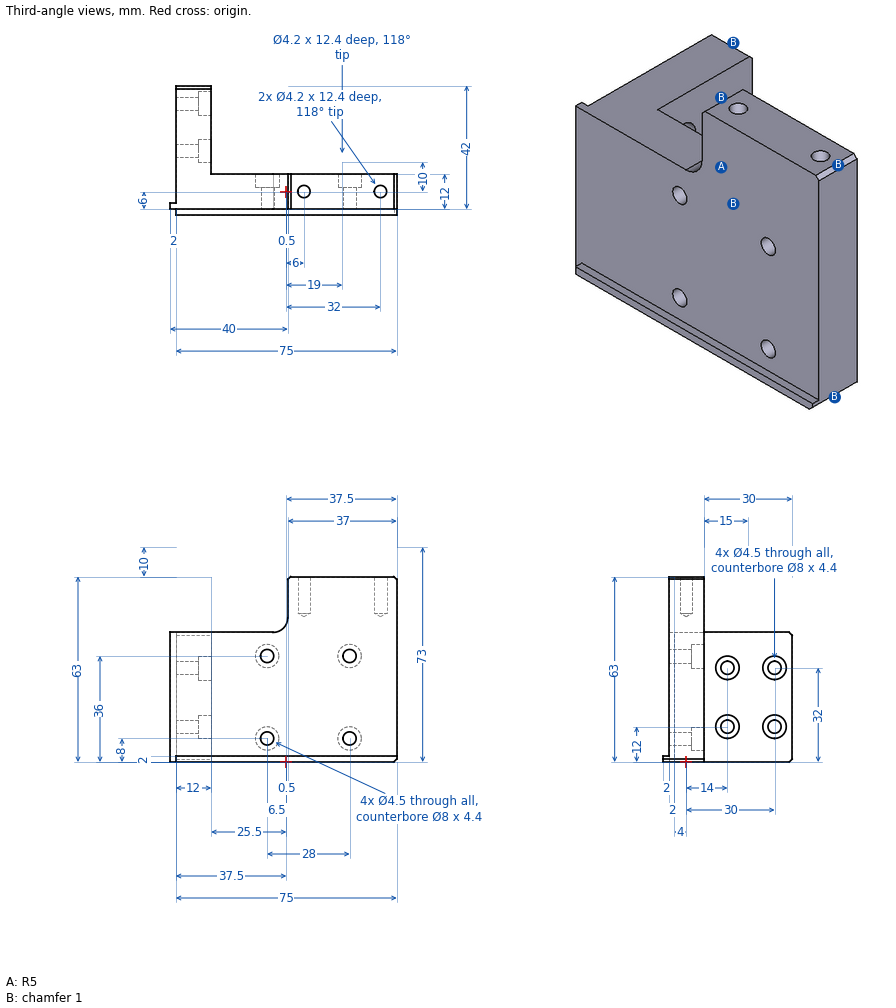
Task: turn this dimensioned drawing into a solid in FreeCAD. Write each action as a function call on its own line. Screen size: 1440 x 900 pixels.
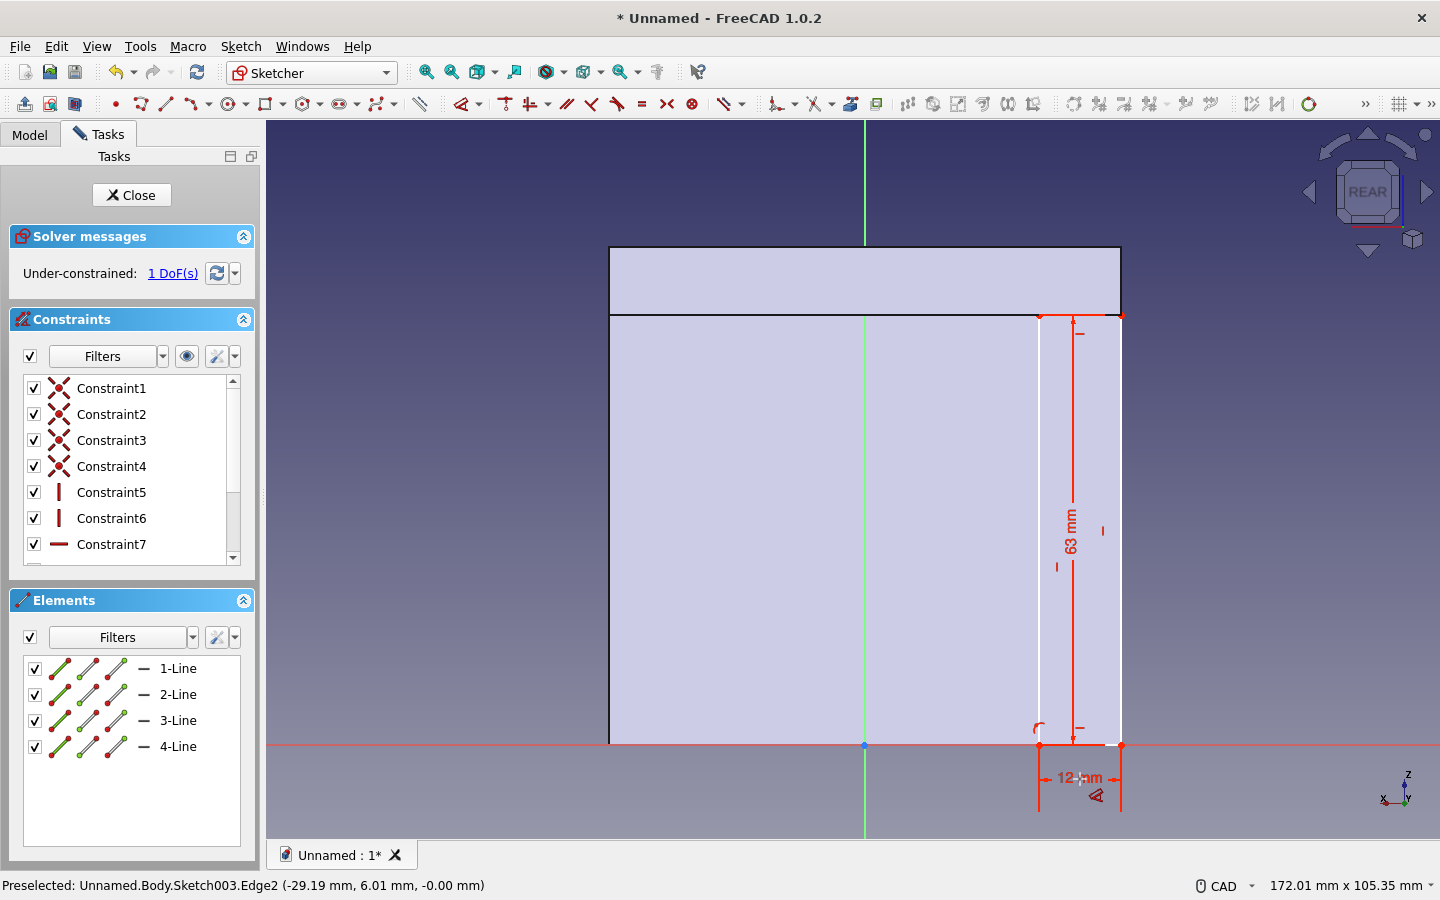
click(1039, 315)
click(952, 779)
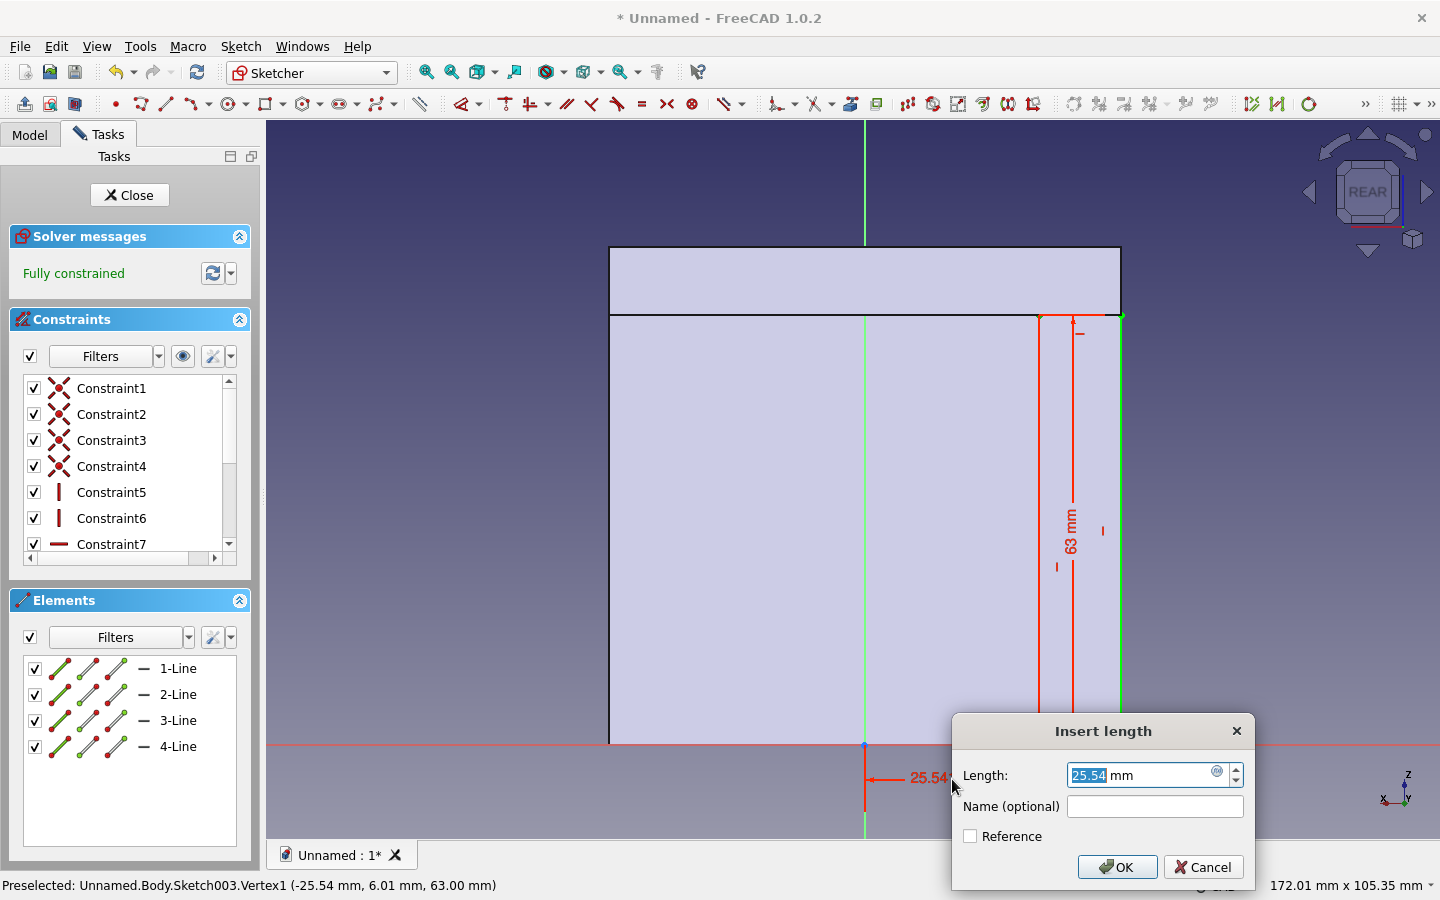
text(25.5)
key(Return)
key(Escape)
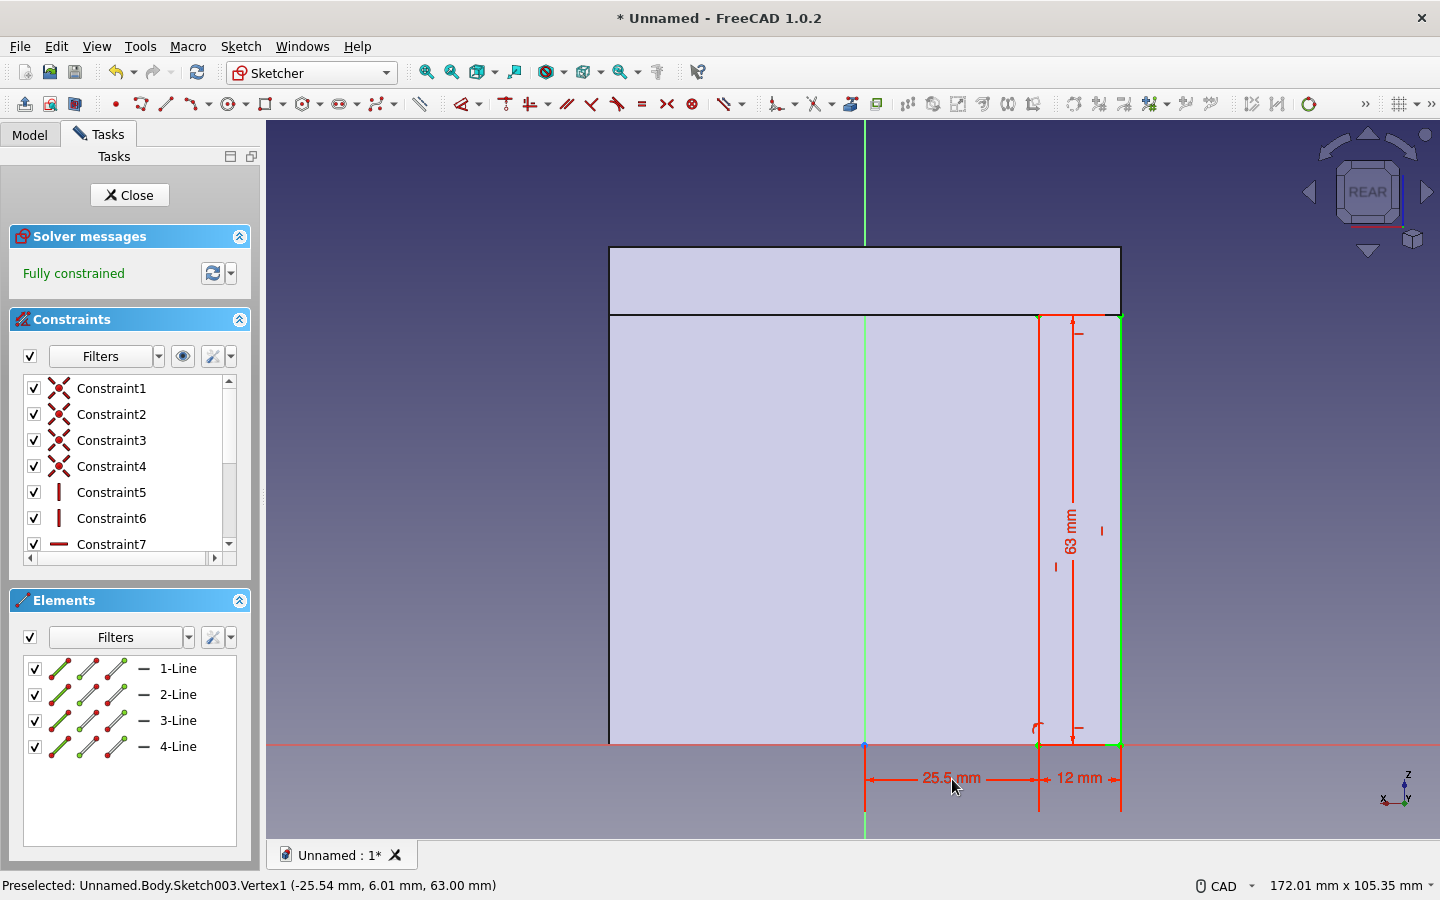
click(130, 195)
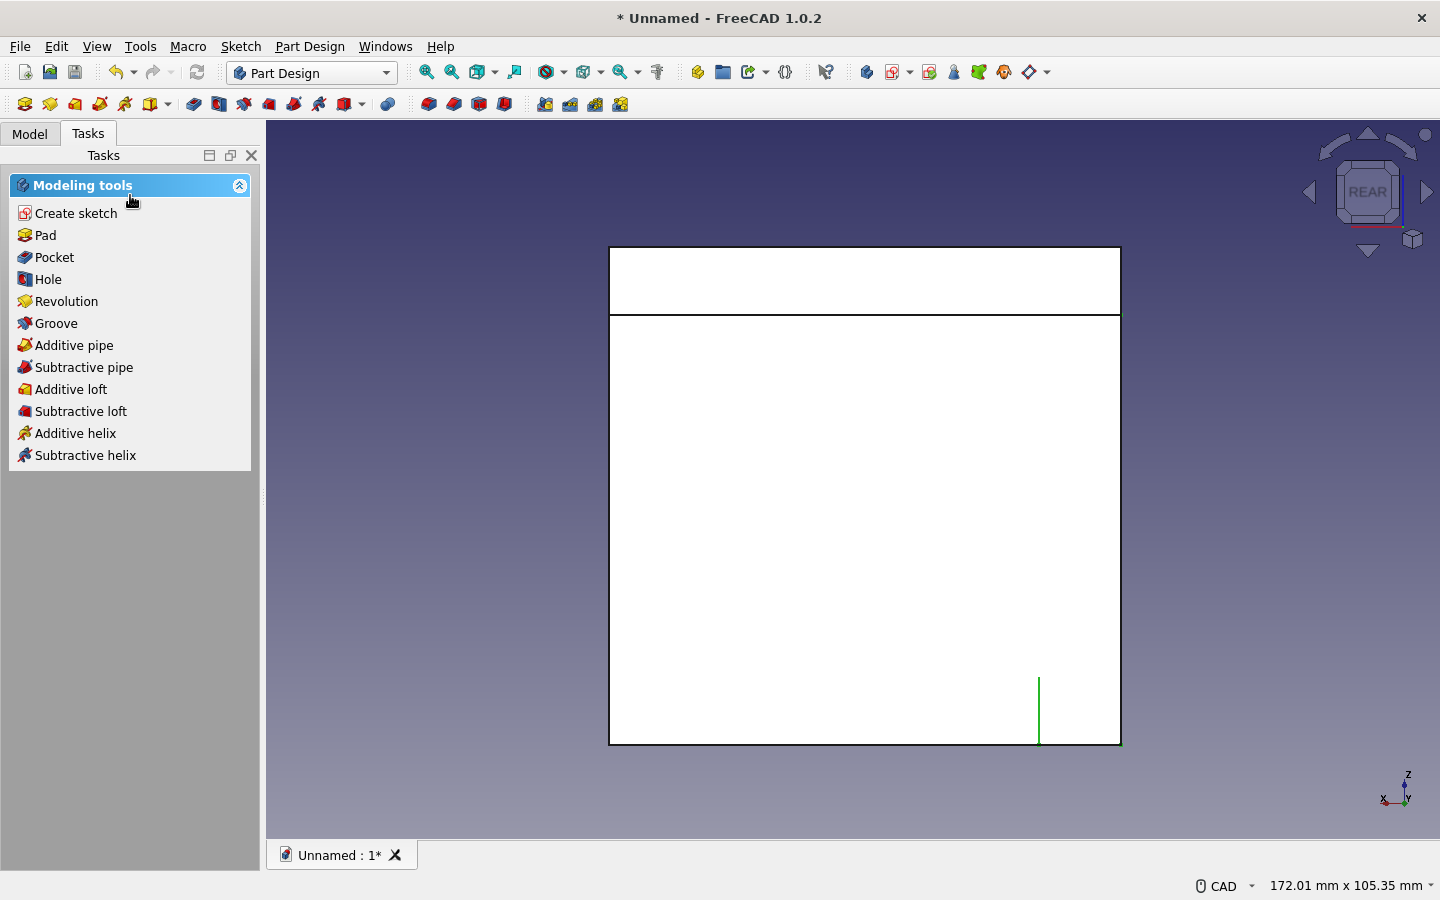
click(25, 104)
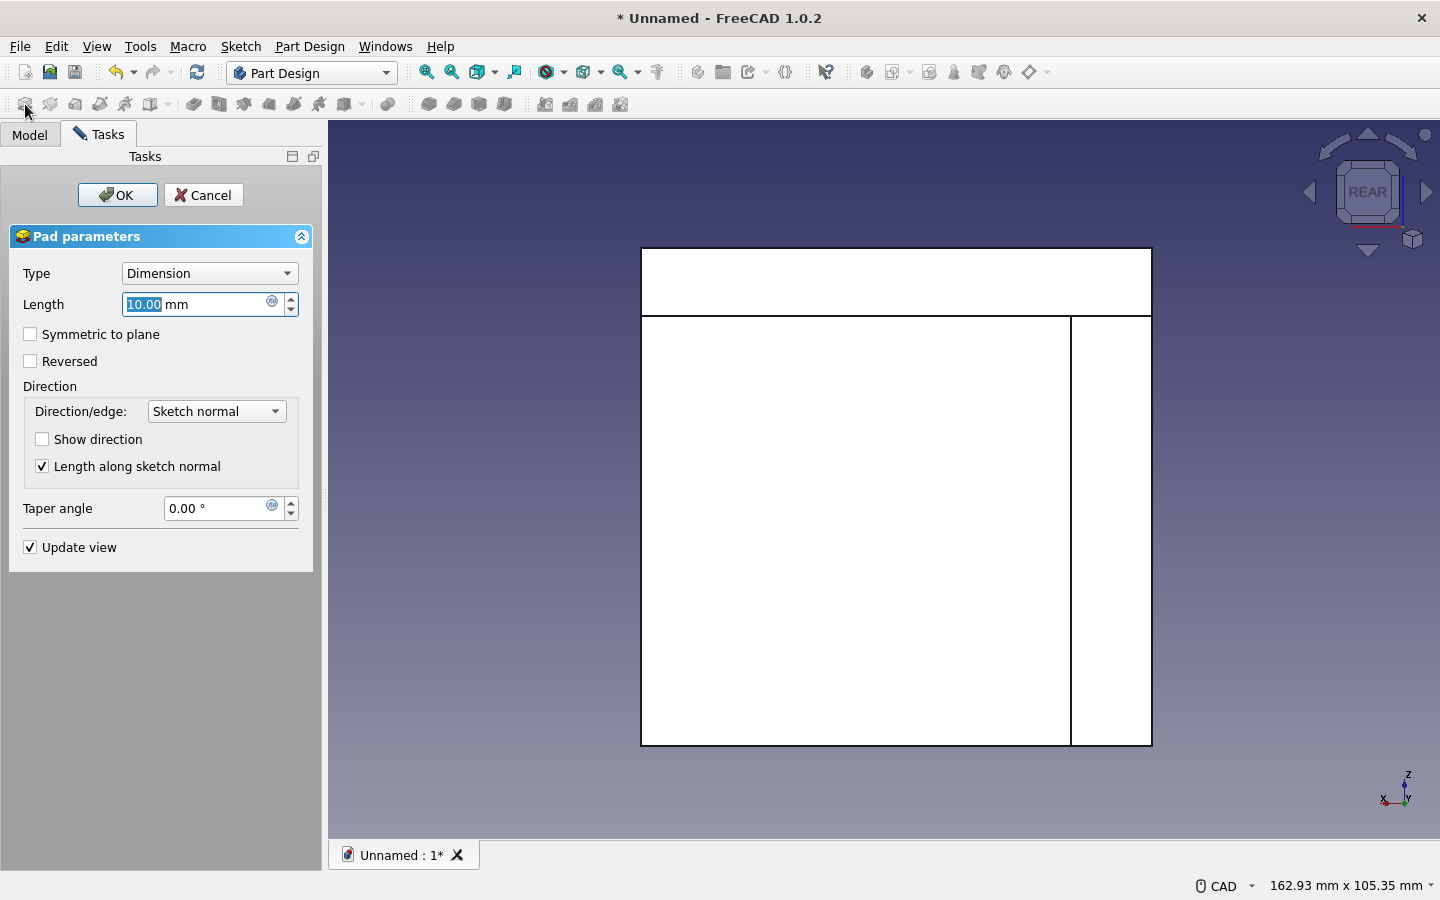
text(30)
key(Tab)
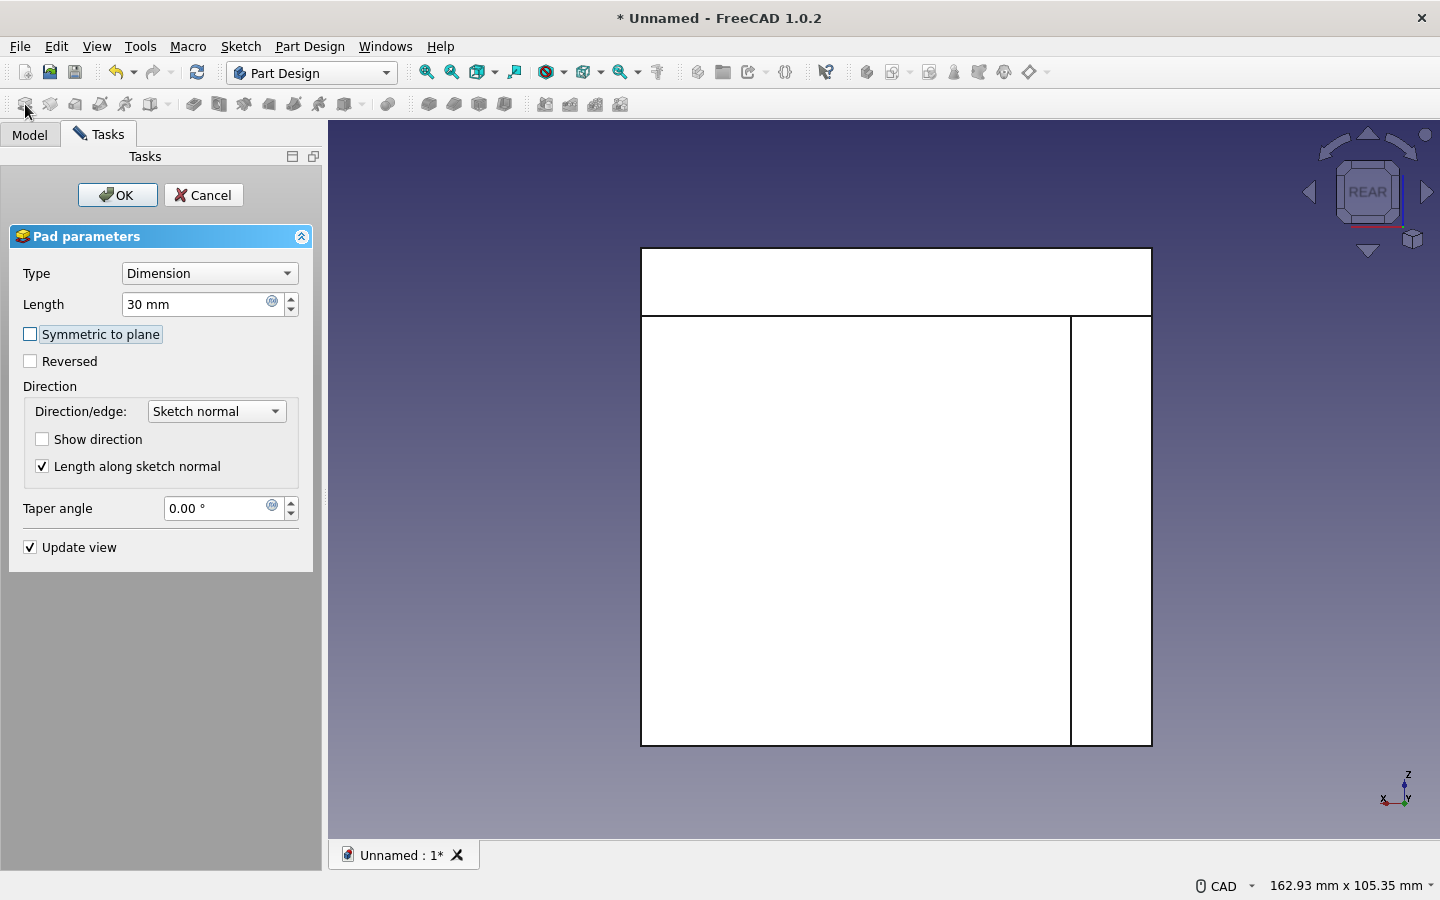
click(118, 195)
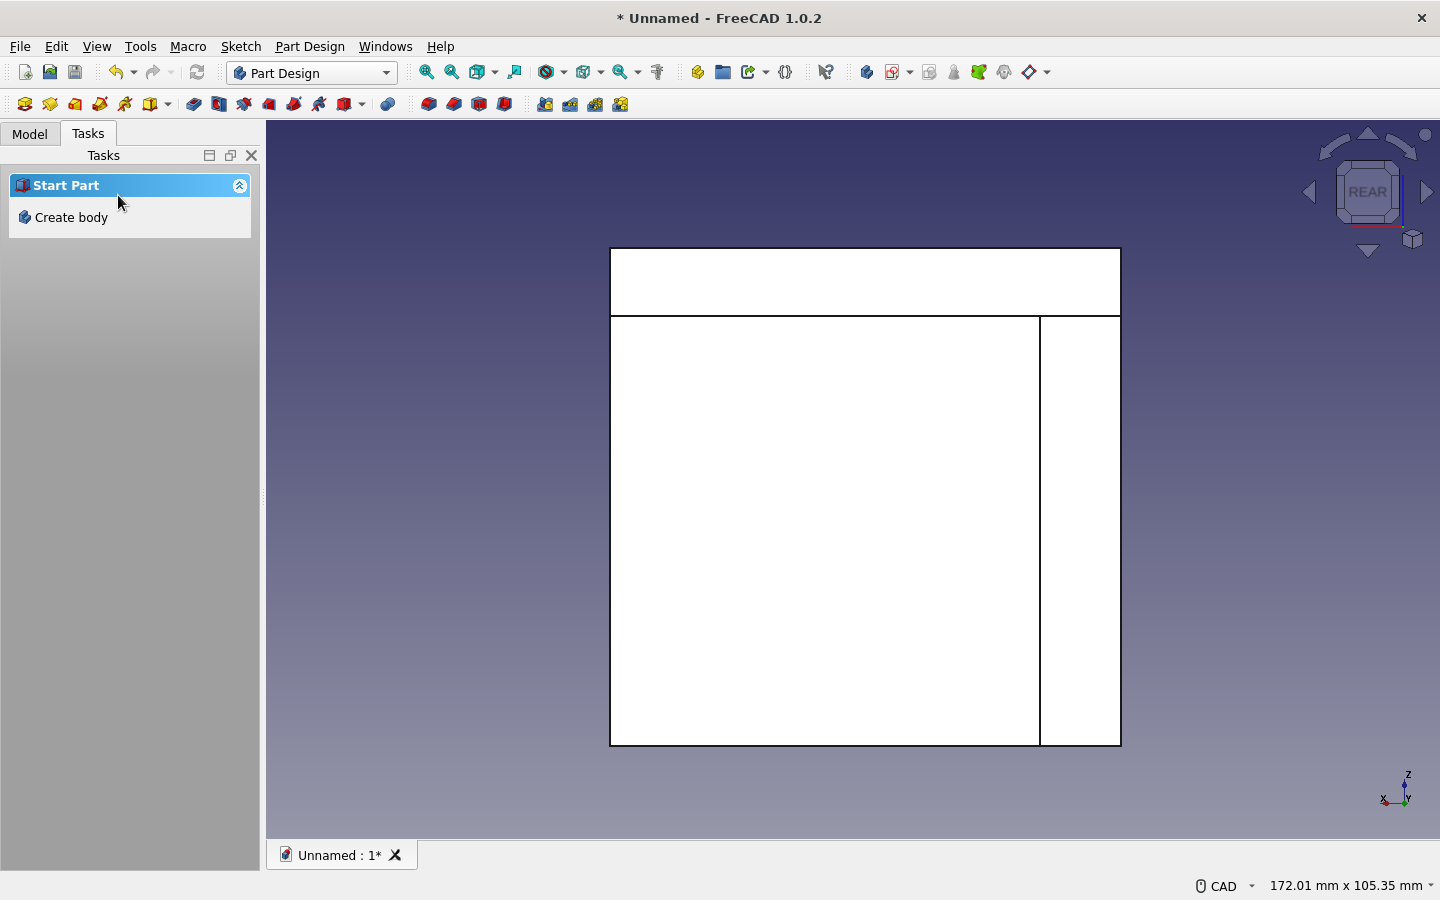
key(6)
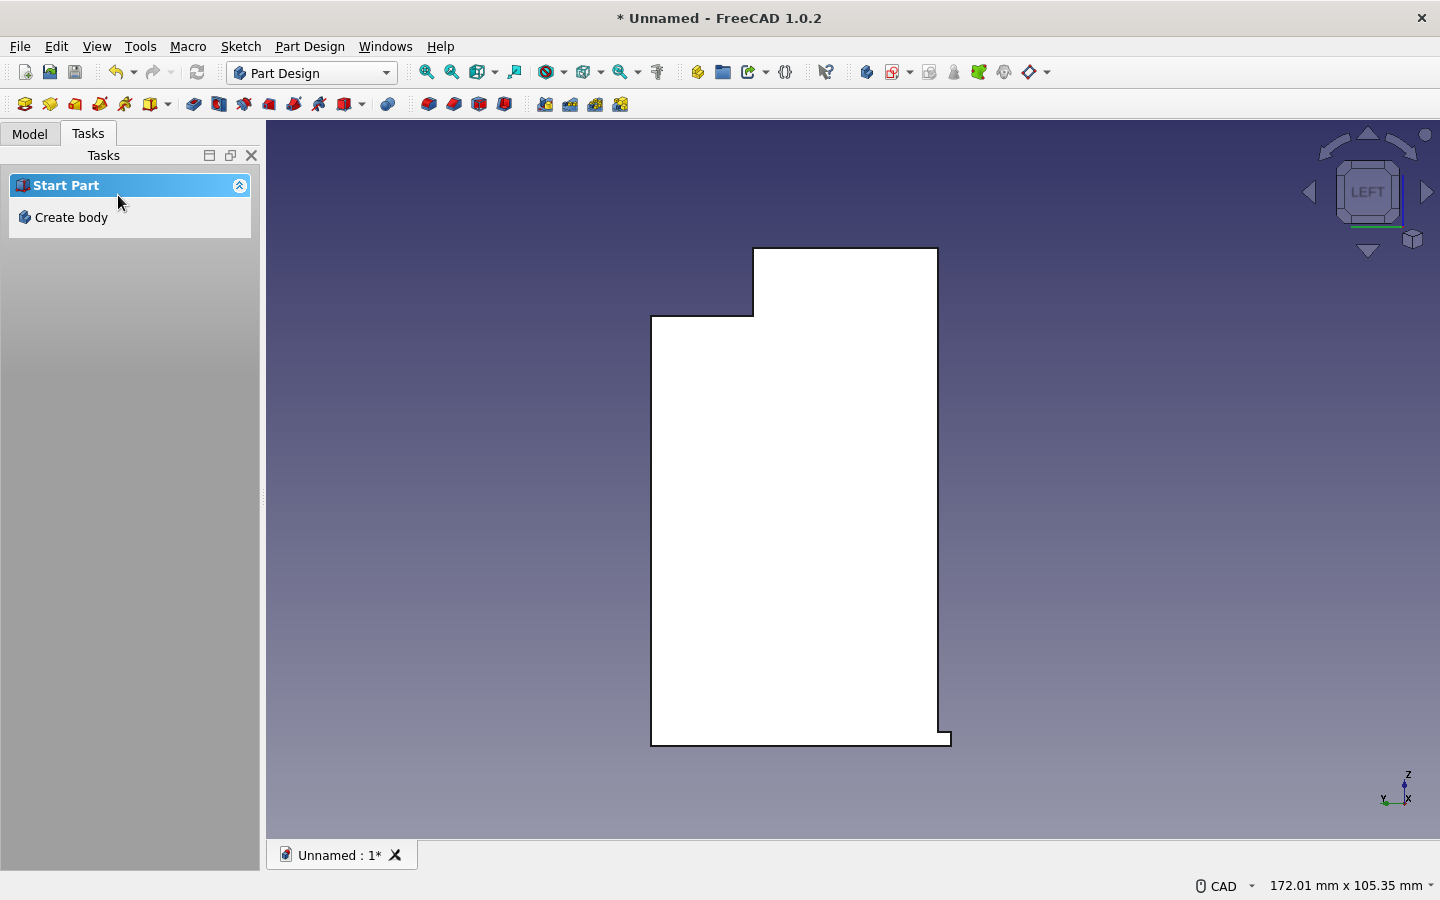
click(801, 496)